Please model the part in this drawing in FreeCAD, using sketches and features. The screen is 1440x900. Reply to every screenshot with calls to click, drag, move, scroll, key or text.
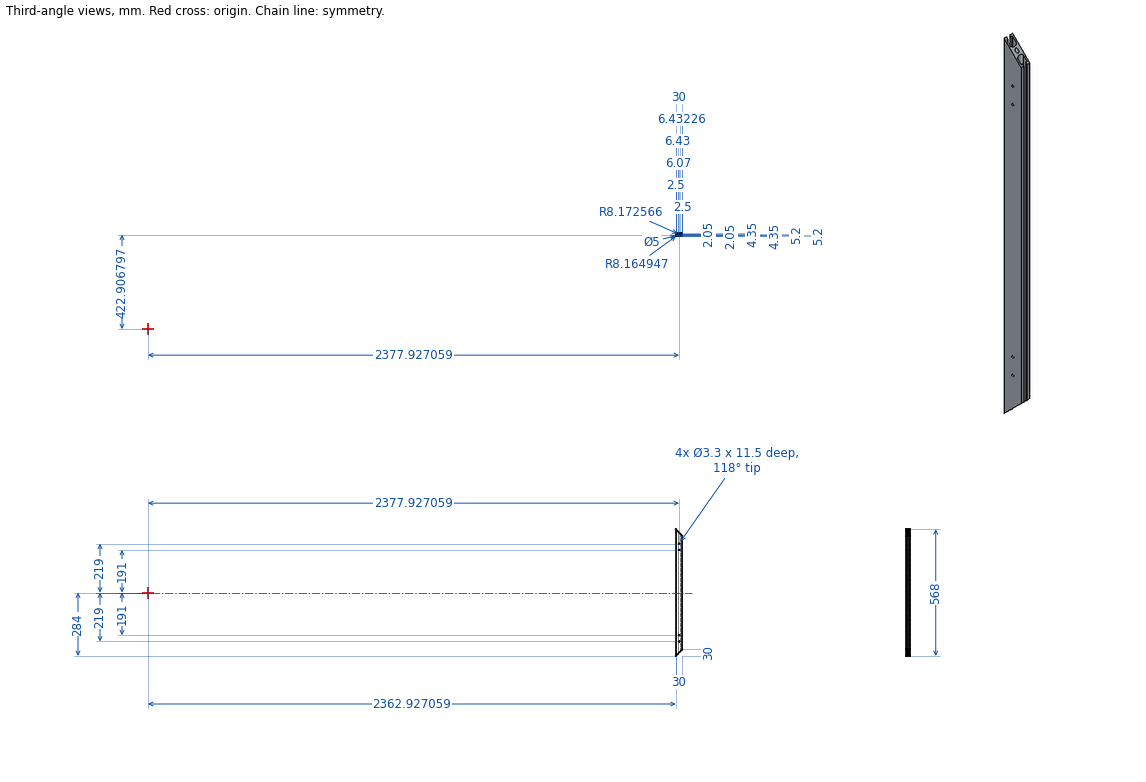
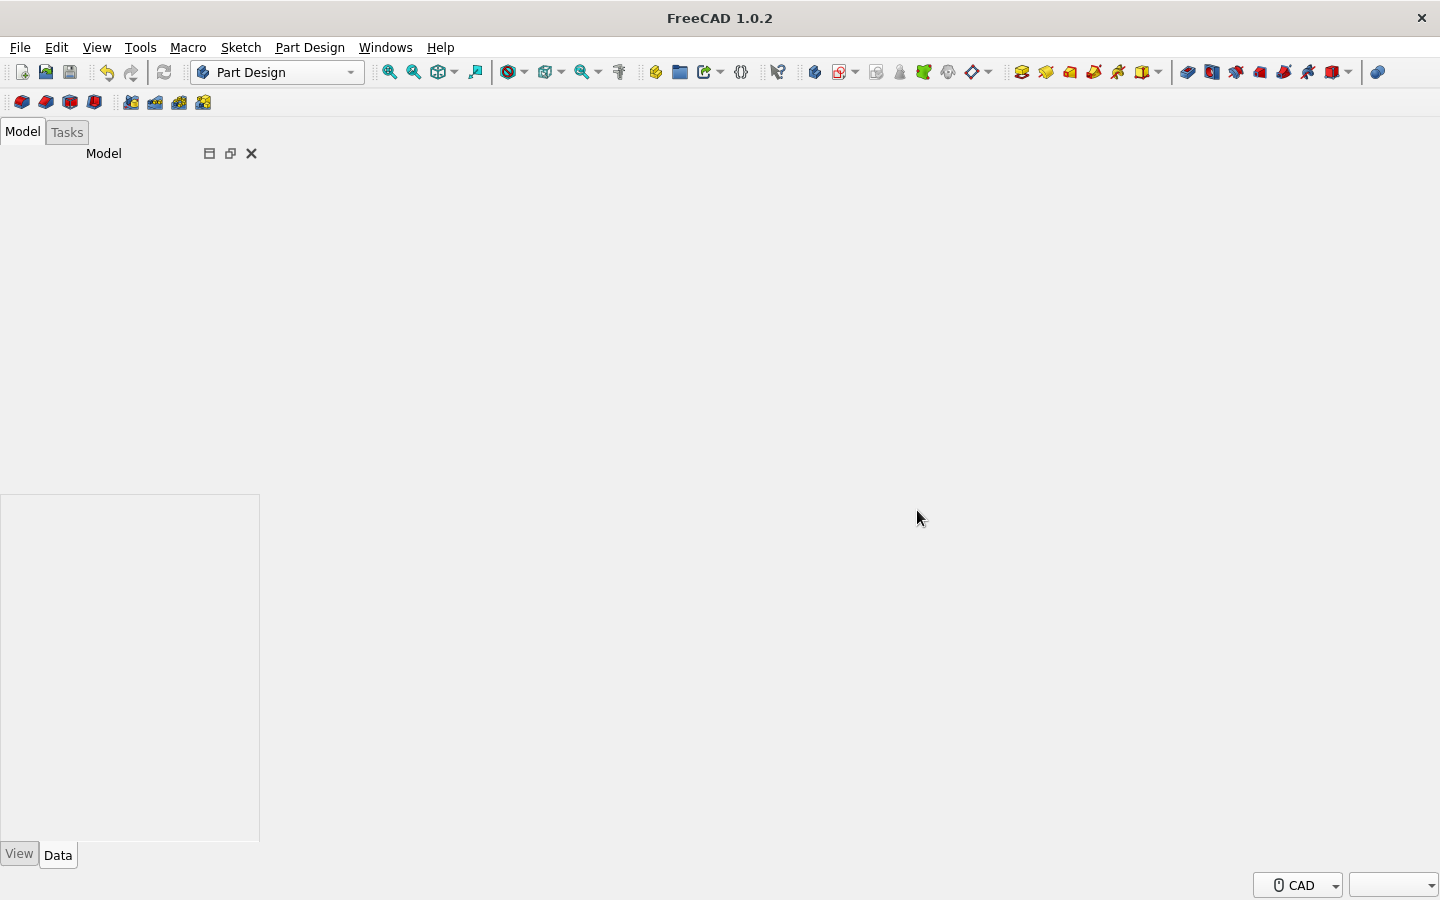
click(22, 72)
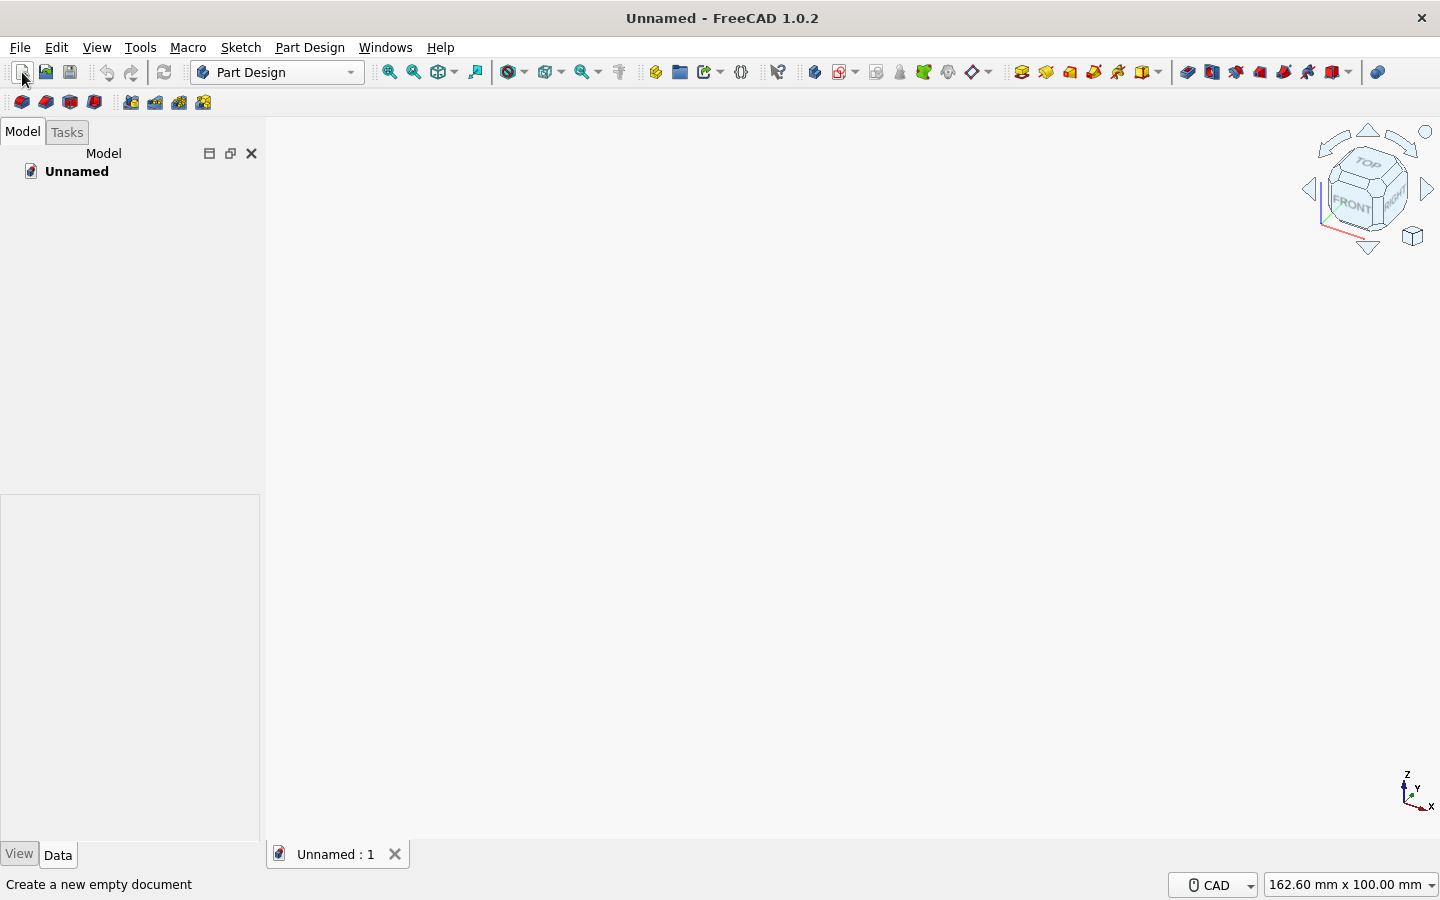
click(840, 72)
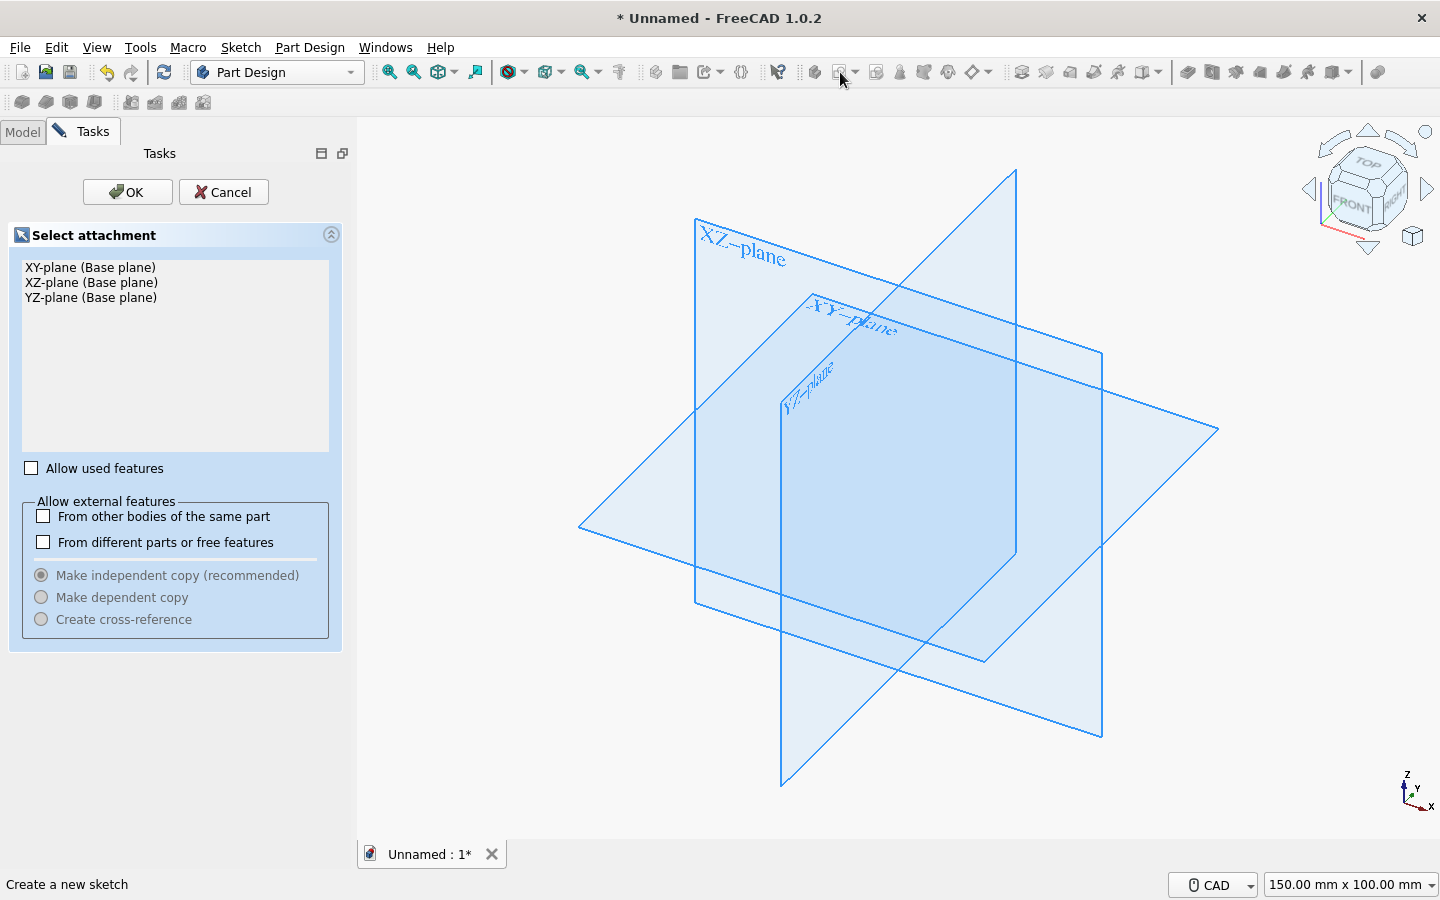
click(82, 268)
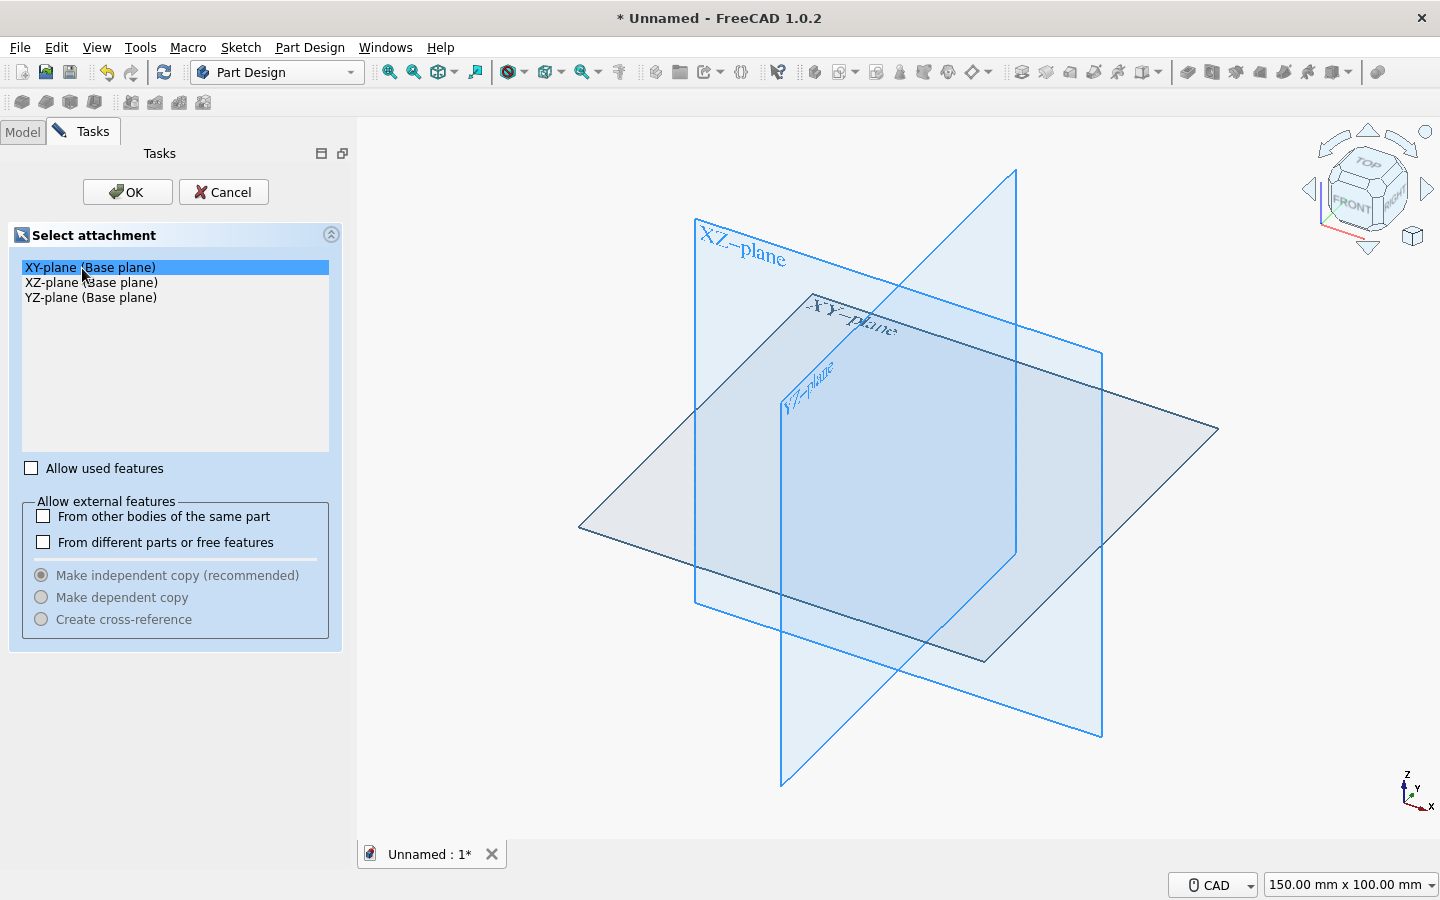
click(128, 192)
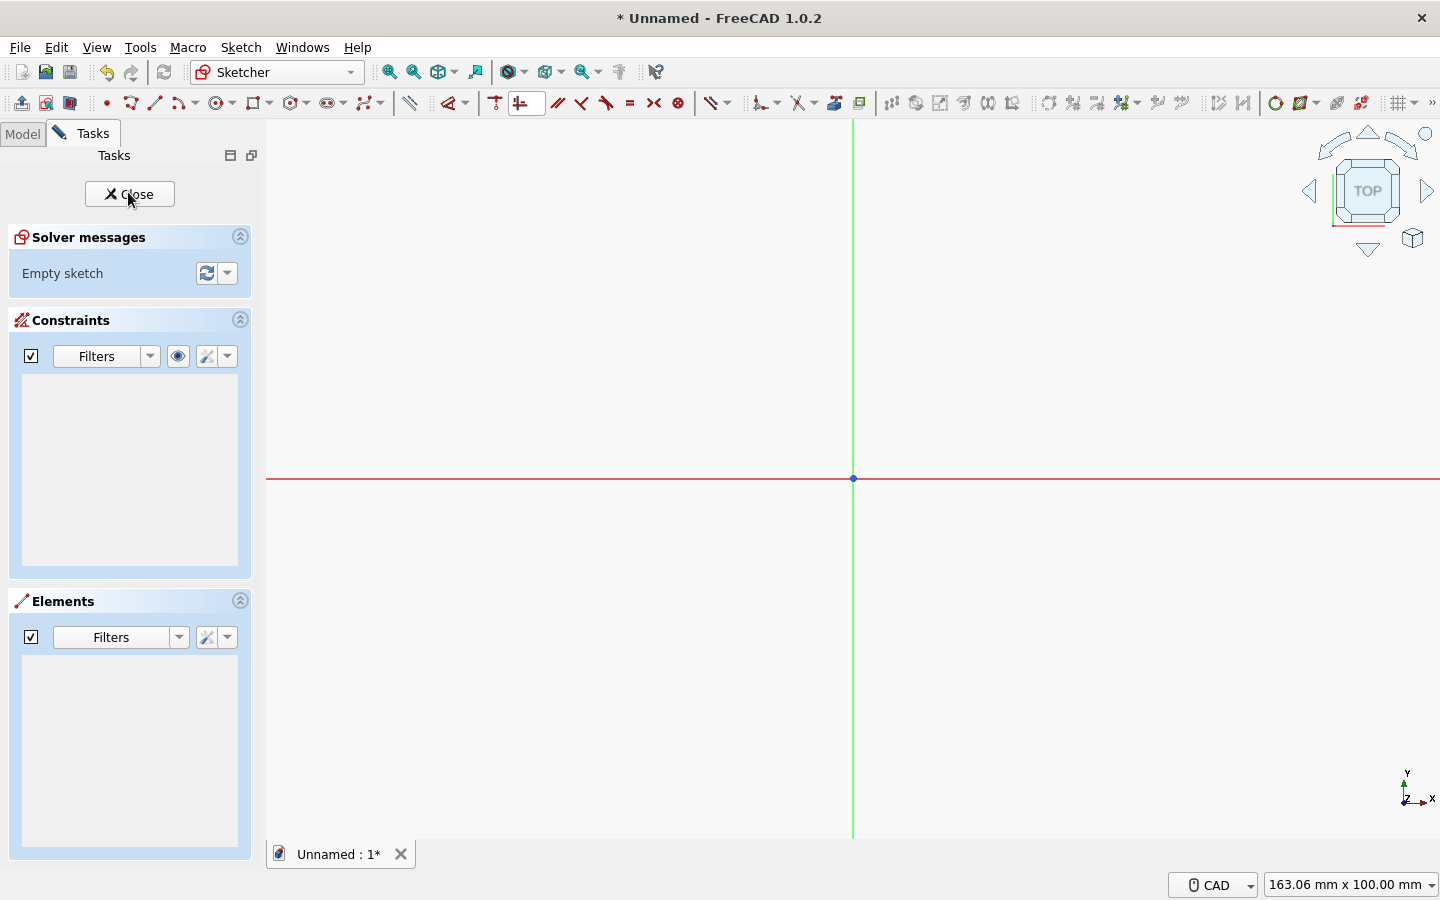
scroll(784, 479, down, 5)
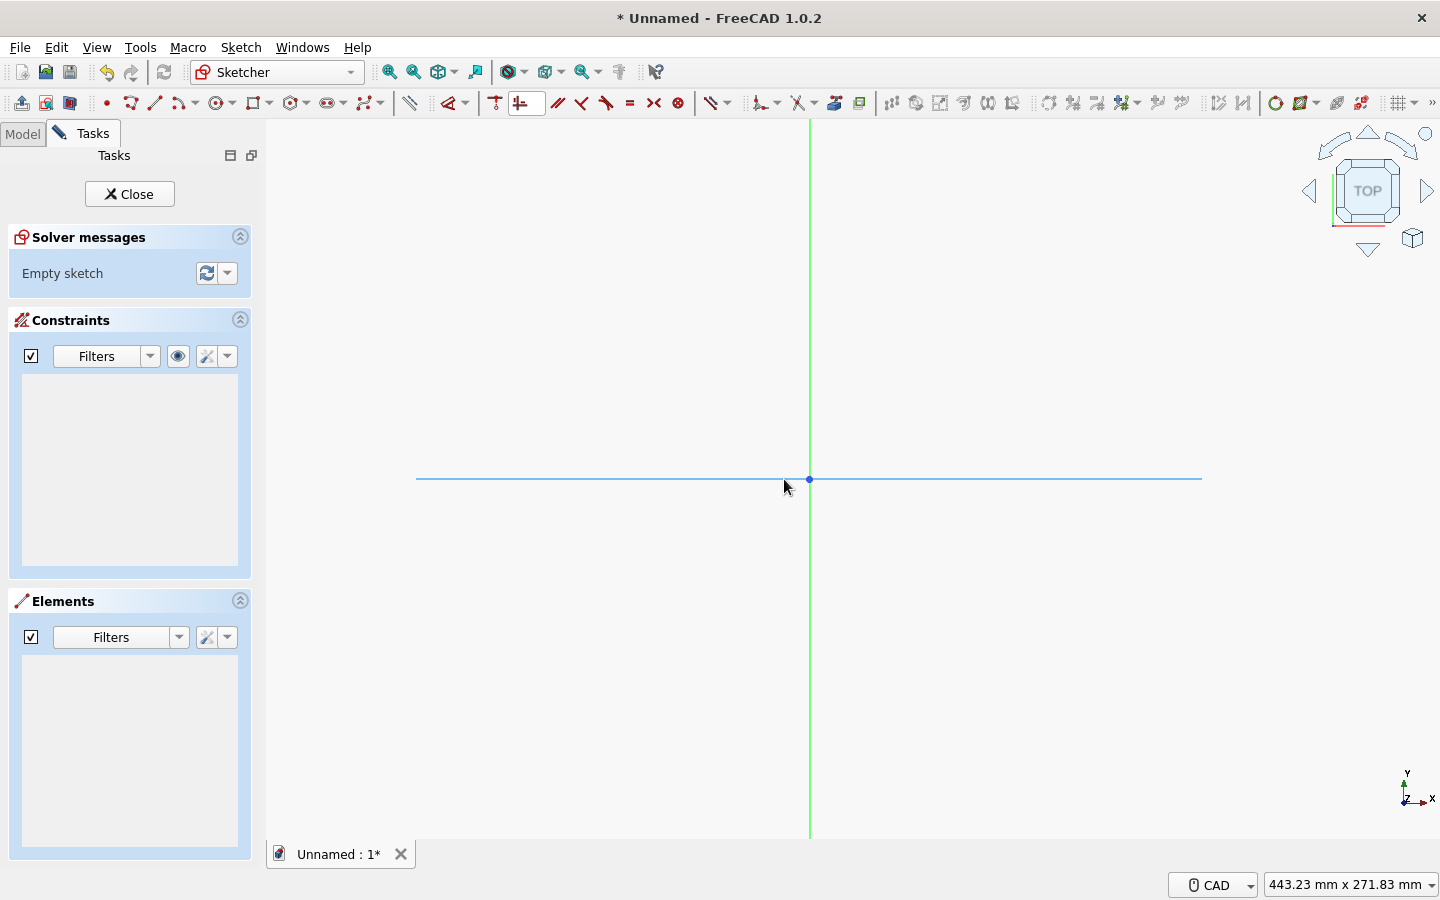
scroll(784, 479, down, 5)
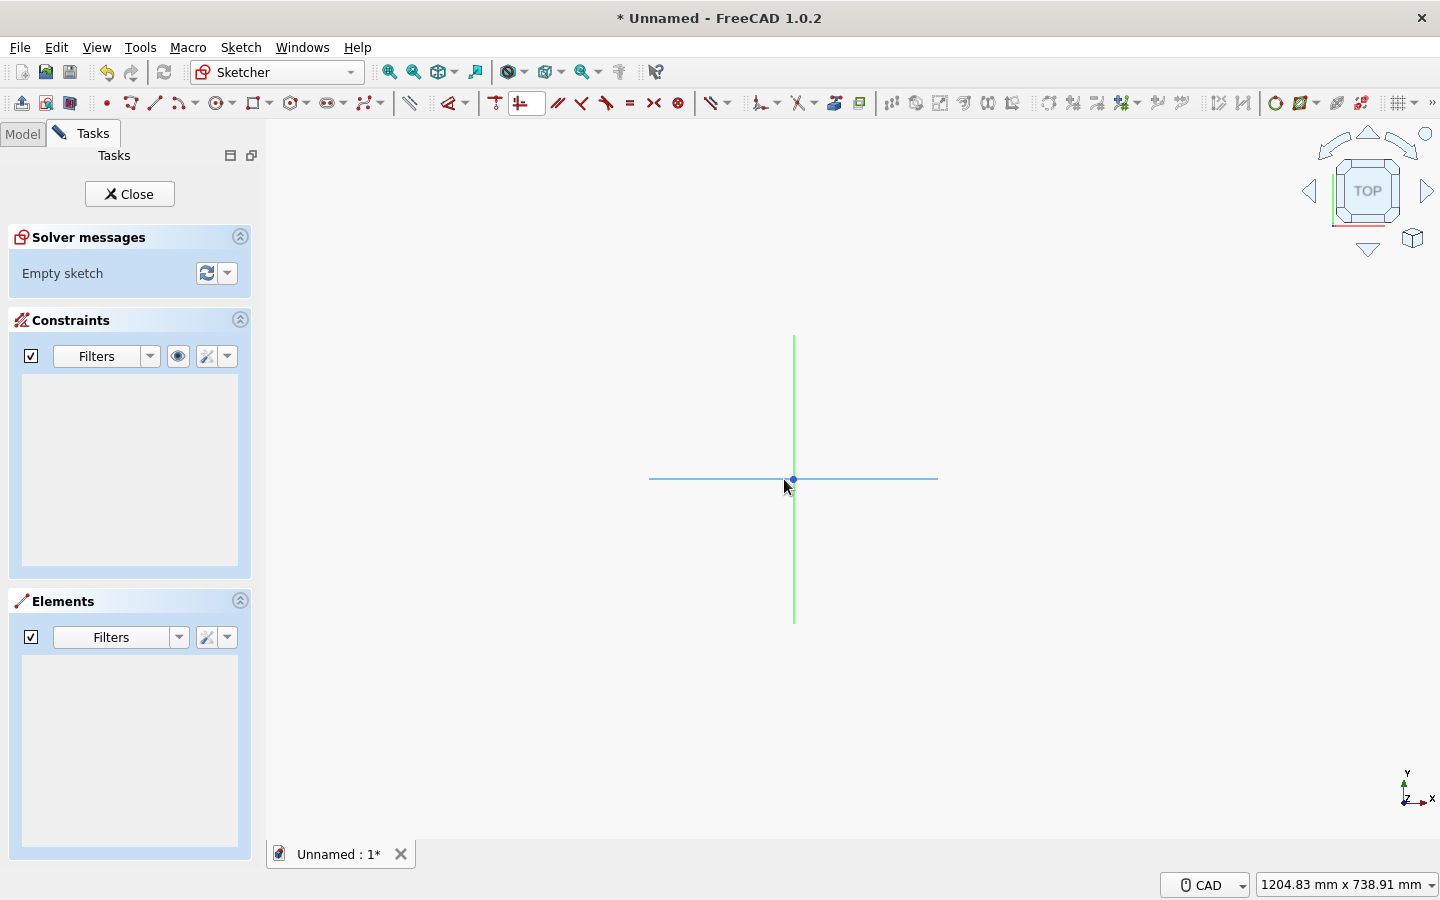
scroll(784, 479, down, 5)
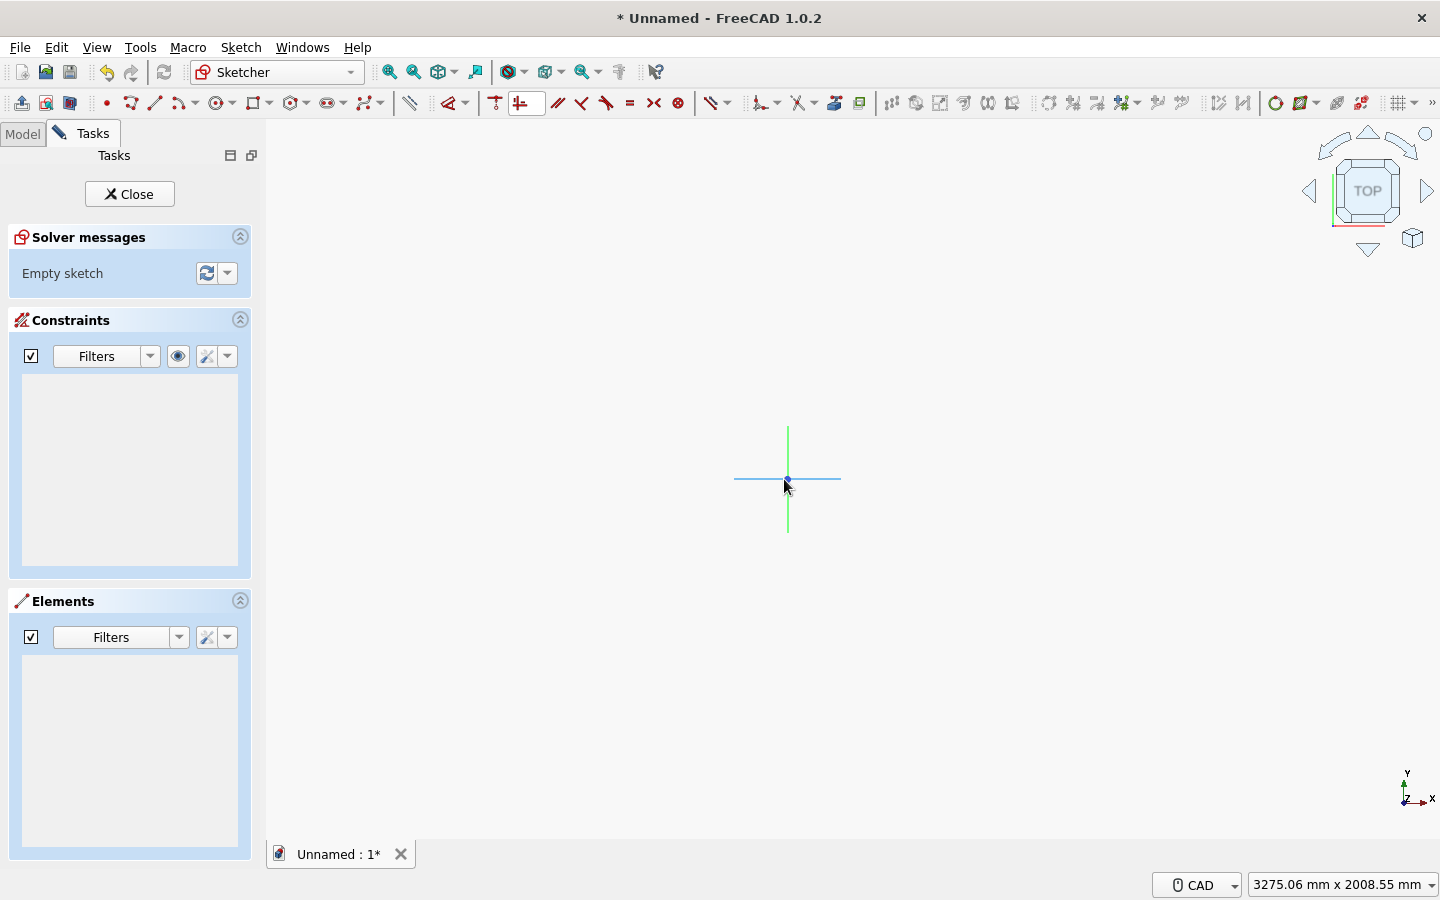
scroll(784, 479, down, 5)